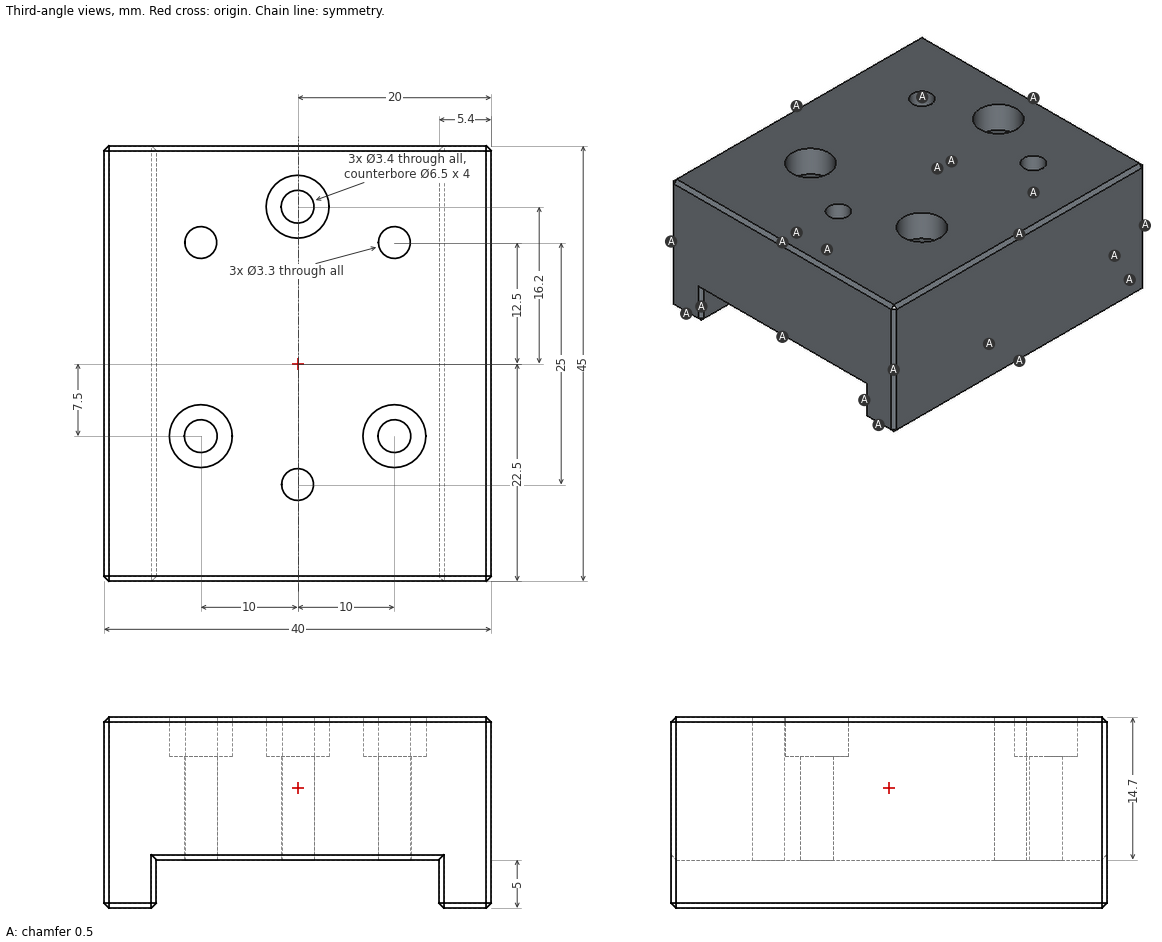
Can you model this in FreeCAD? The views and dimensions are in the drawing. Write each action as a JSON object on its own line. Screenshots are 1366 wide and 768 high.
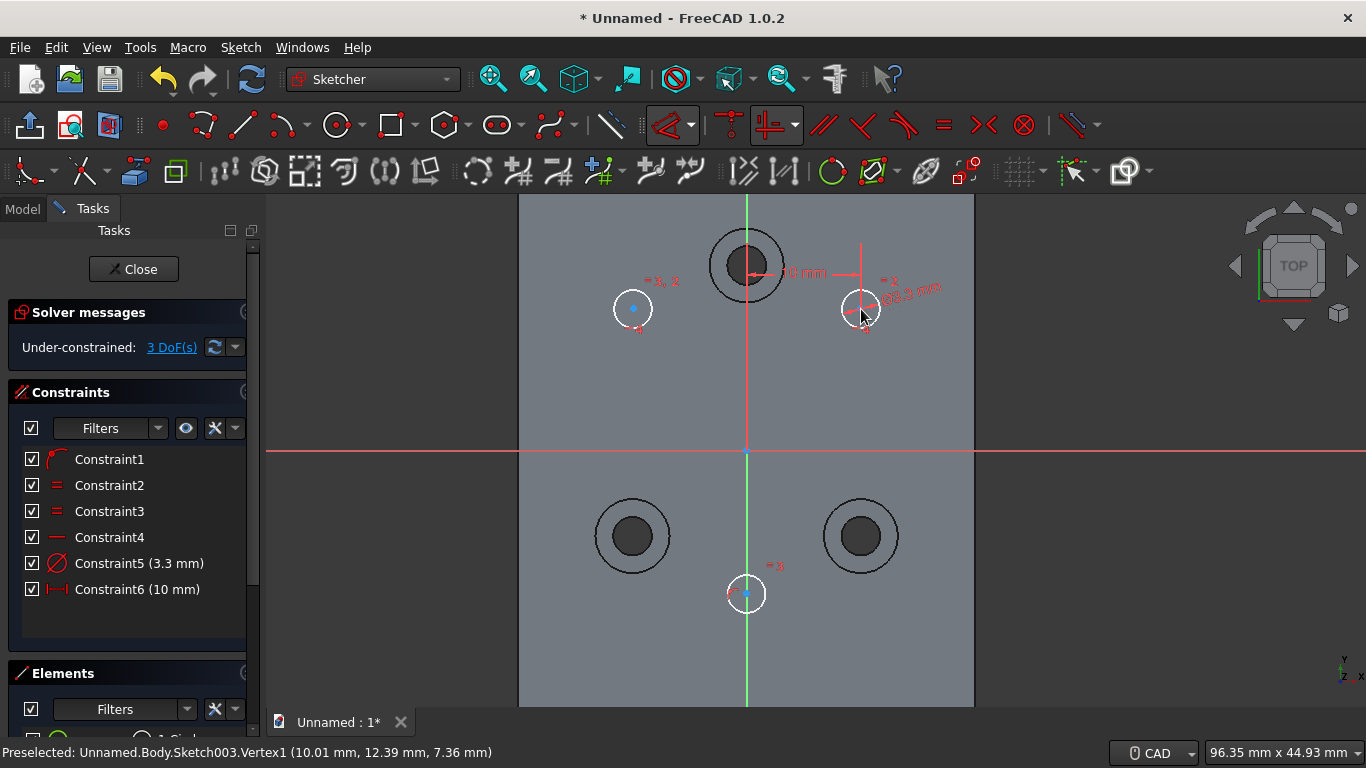
{"action": "left_click", "coordinate": [633, 309]}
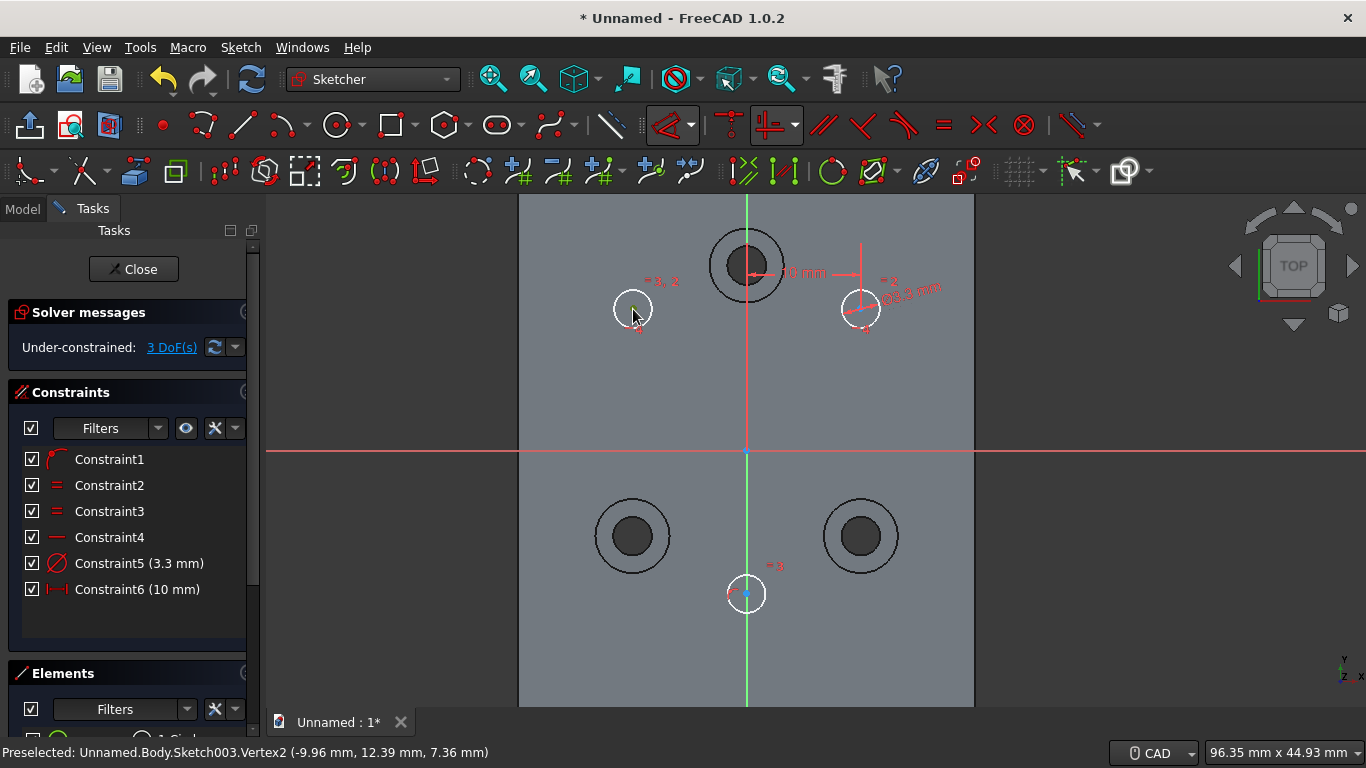
{"action": "key", "text": "l"}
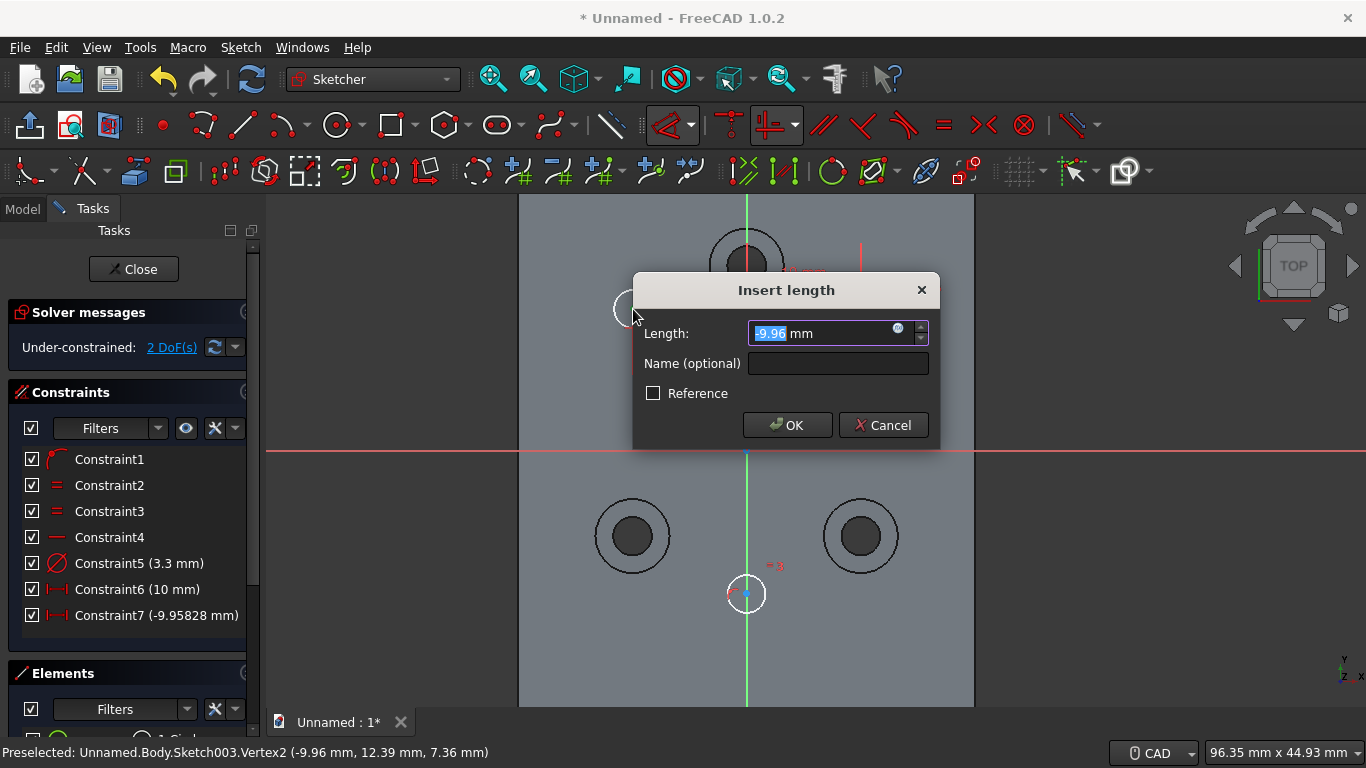
{"action": "type", "text": "-10"}
{"action": "key", "text": "Return"}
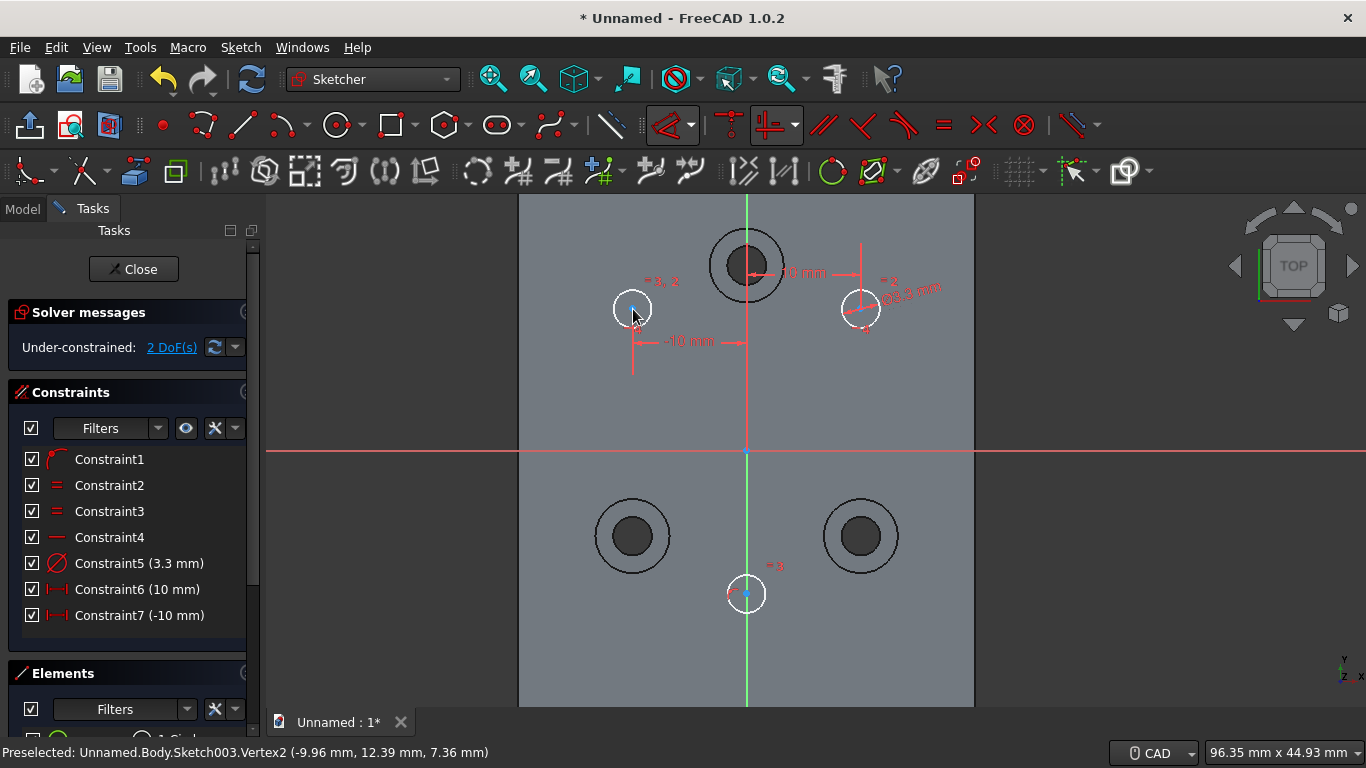
{"action": "left_click", "coordinate": [861, 309]}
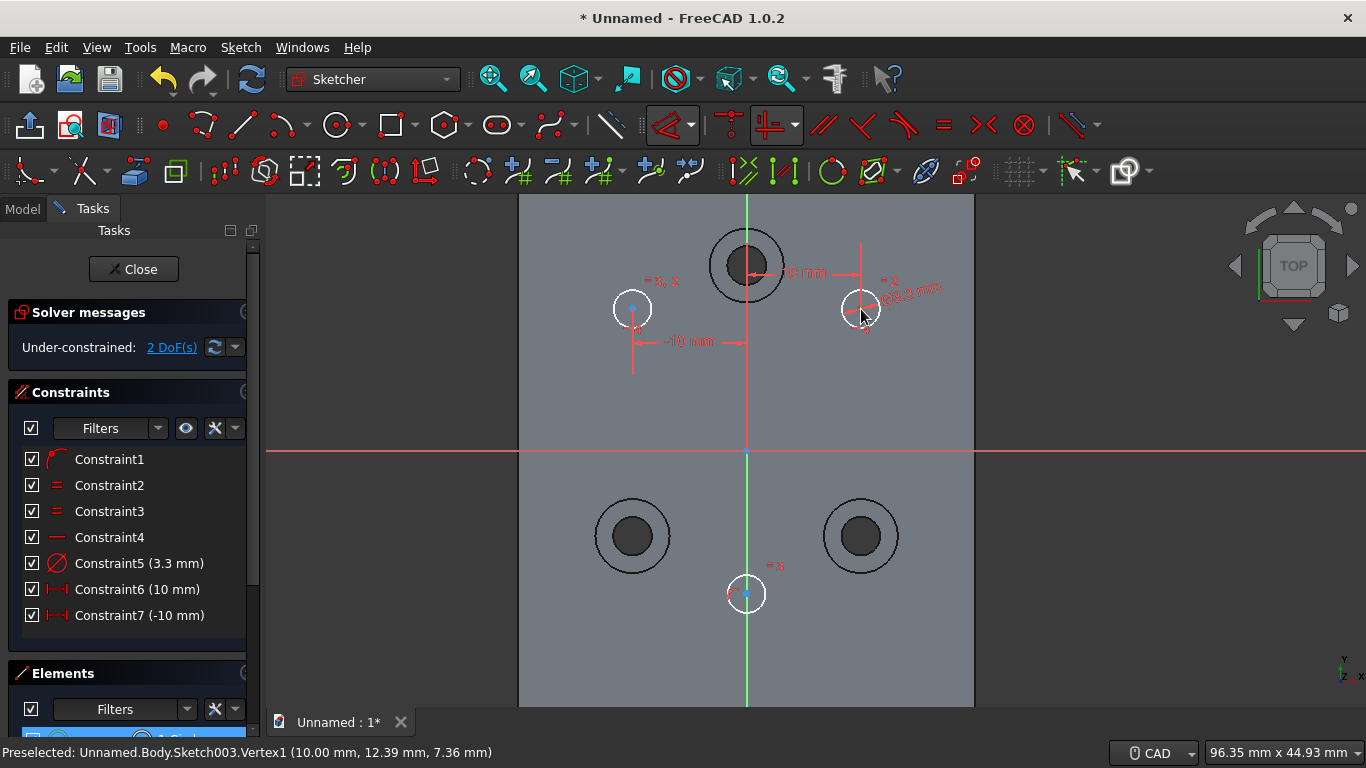
{"action": "left_click", "coordinate": [747, 594]}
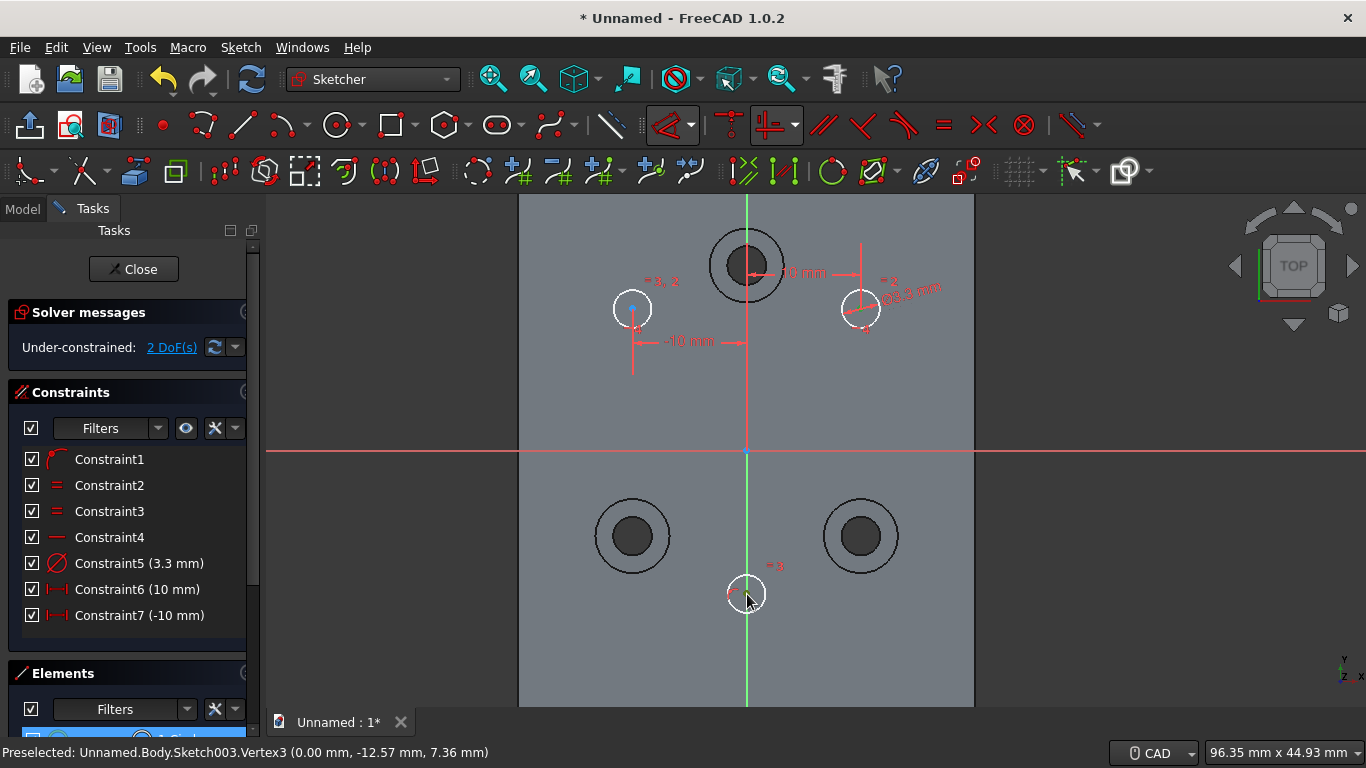
{"action": "key", "text": "i"}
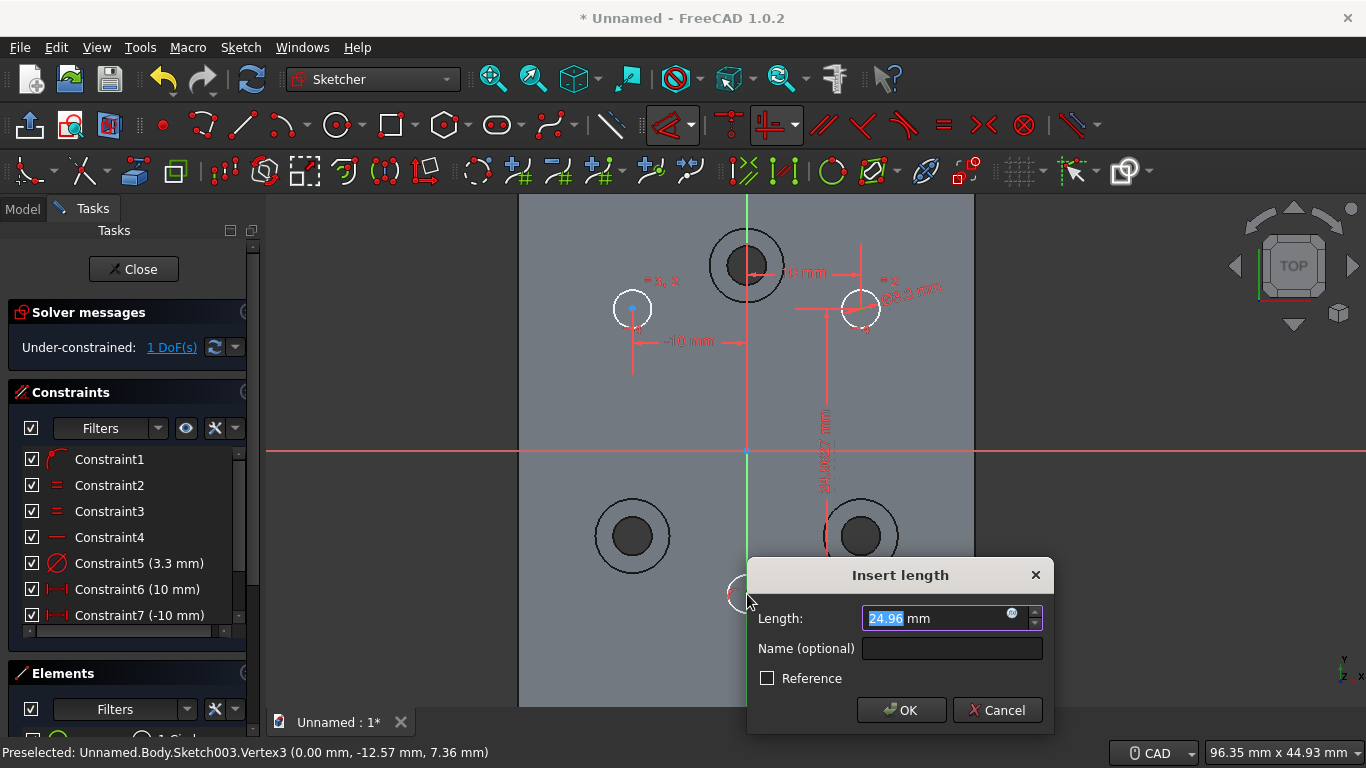
{"action": "type", "text": "25"}
{"action": "key", "text": "Return"}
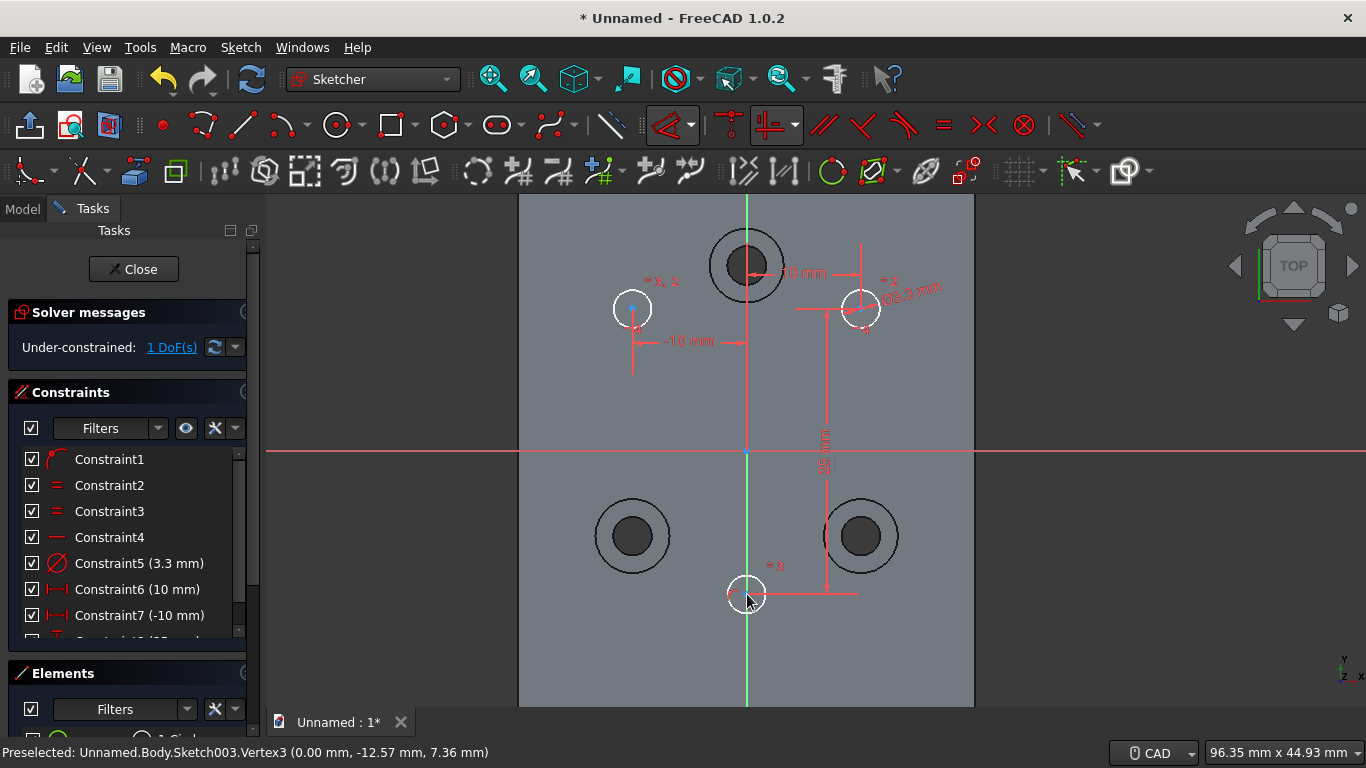
{"action": "left_click", "coordinate": [861, 309]}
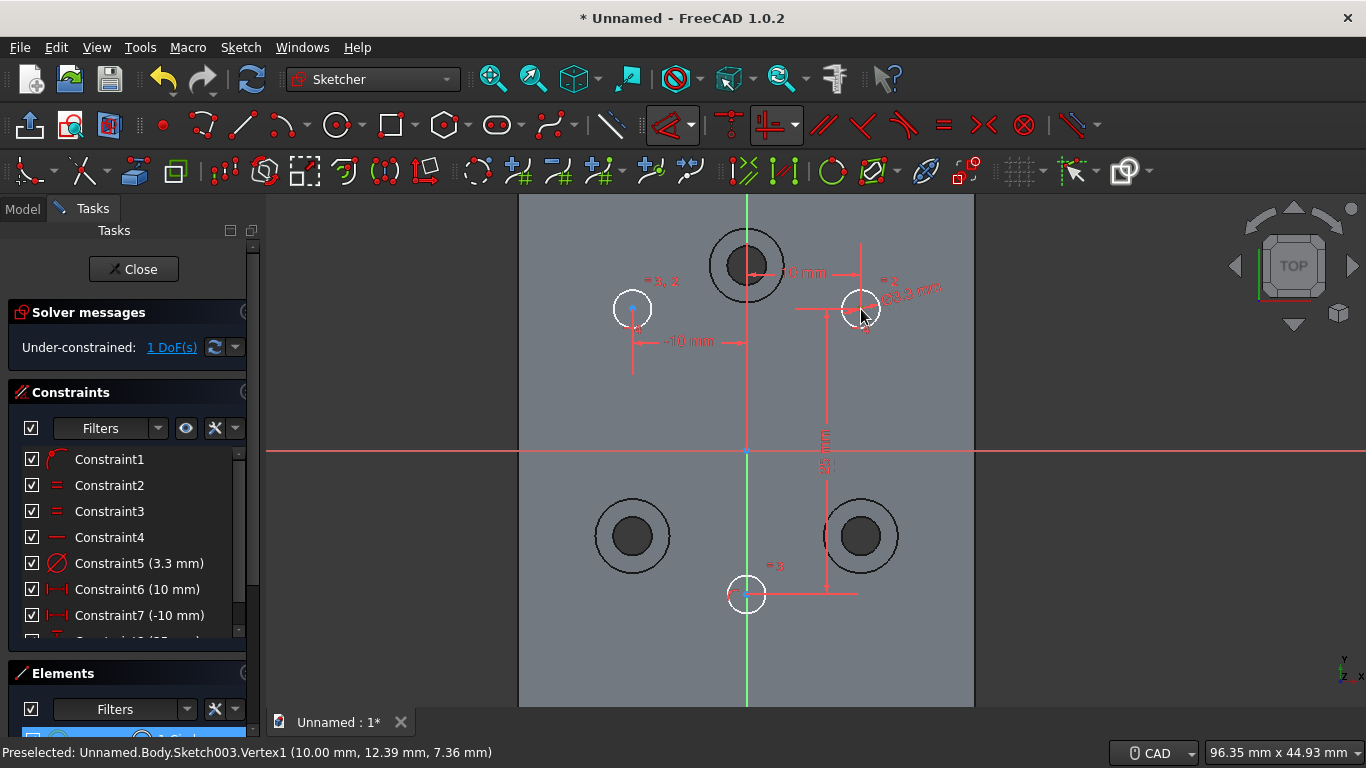
{"action": "left_click", "coordinate": [694, 126]}